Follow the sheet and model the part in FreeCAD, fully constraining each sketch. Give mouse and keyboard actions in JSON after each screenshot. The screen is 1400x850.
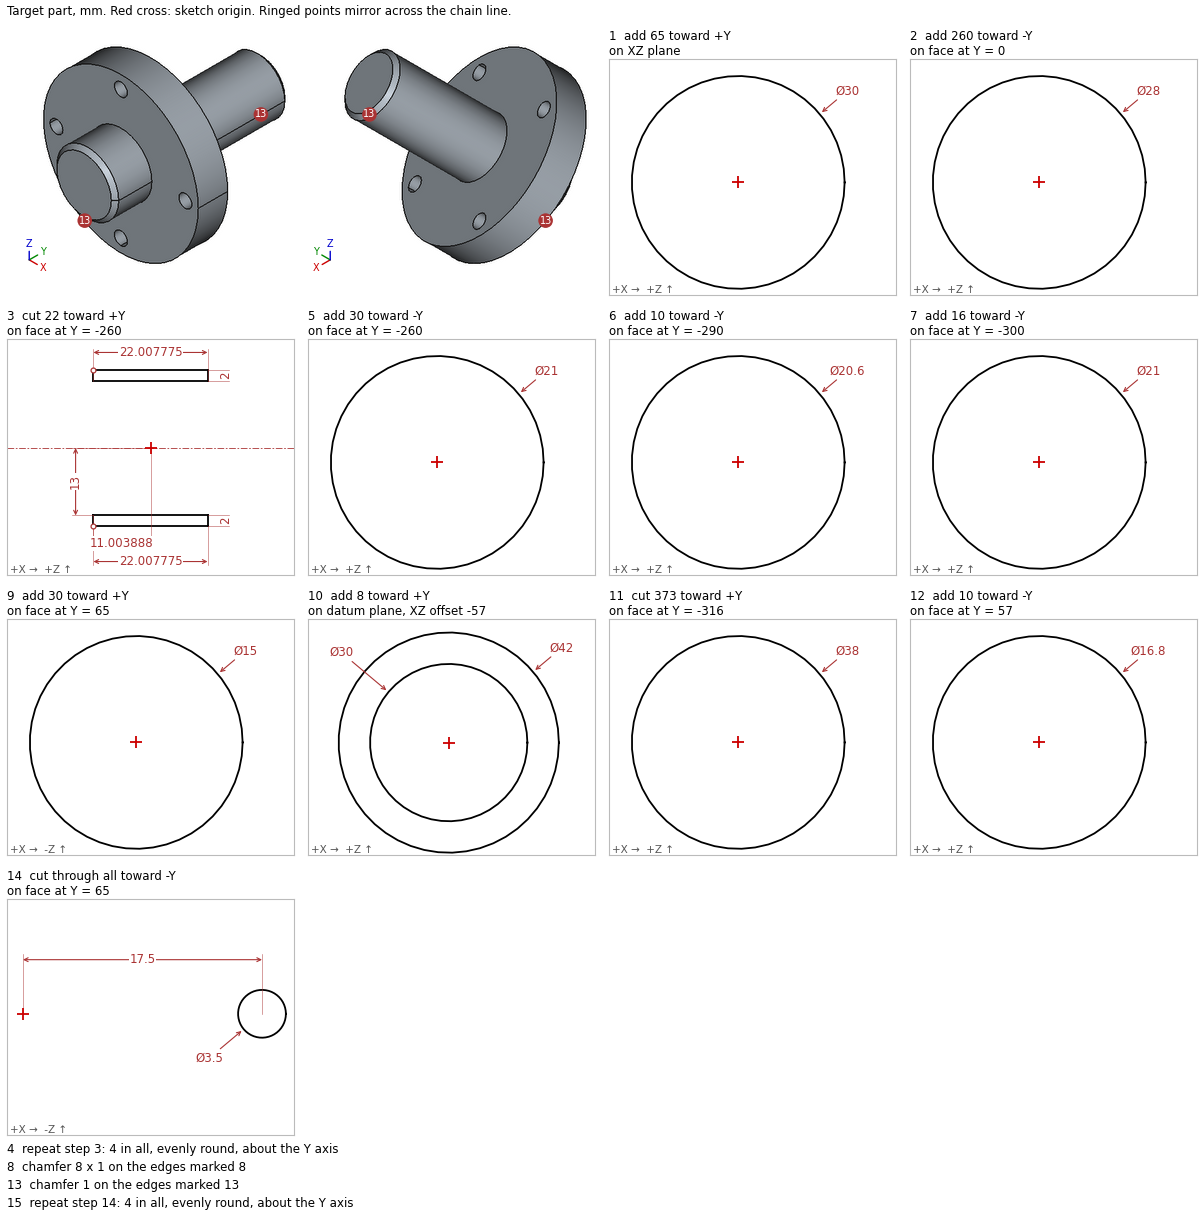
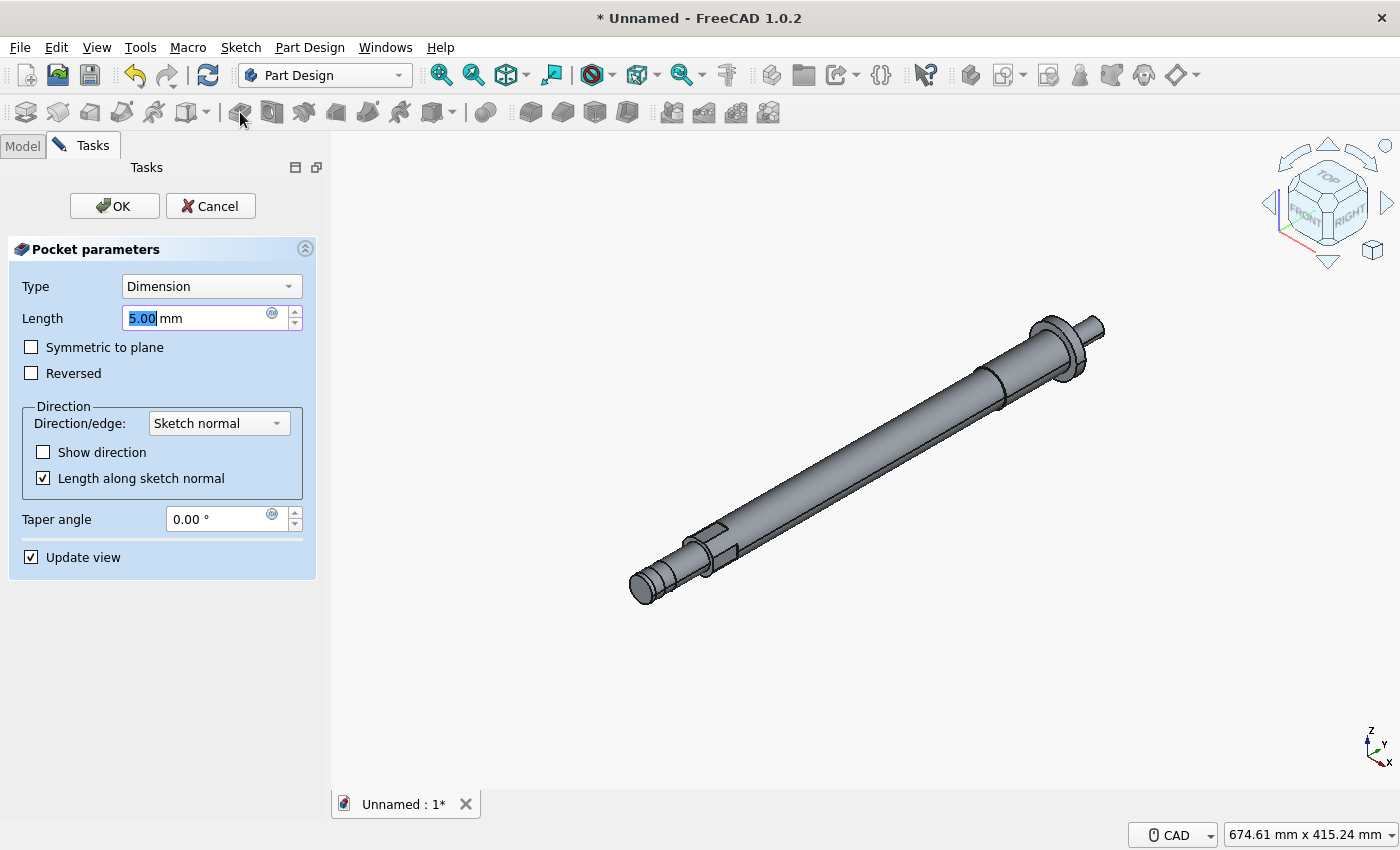
{"action": "type", "text": "373"}
{"action": "key", "text": "Tab"}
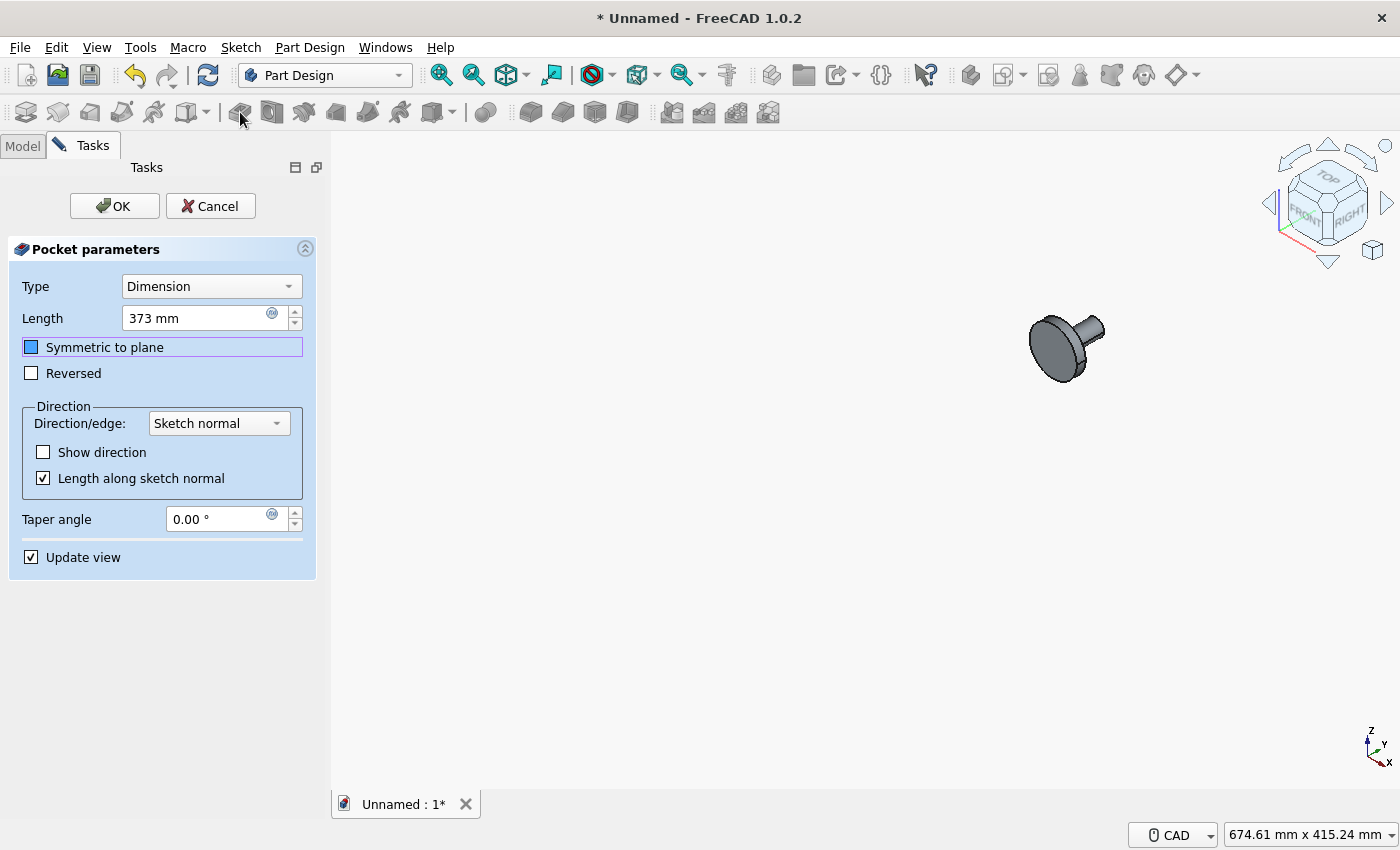
{"action": "left_click", "coordinate": [115, 206]}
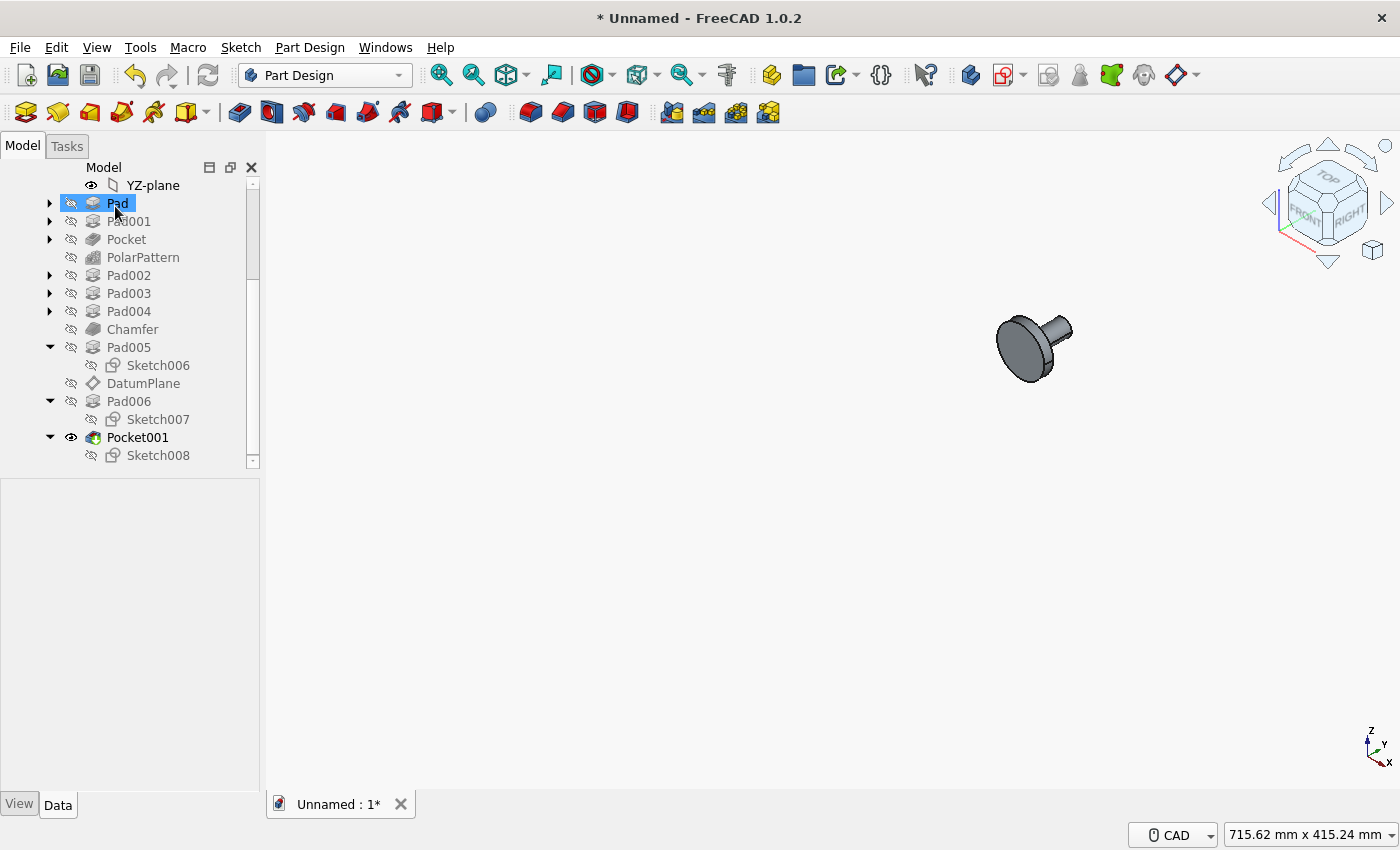
{"action": "left_click", "coordinate": [442, 76]}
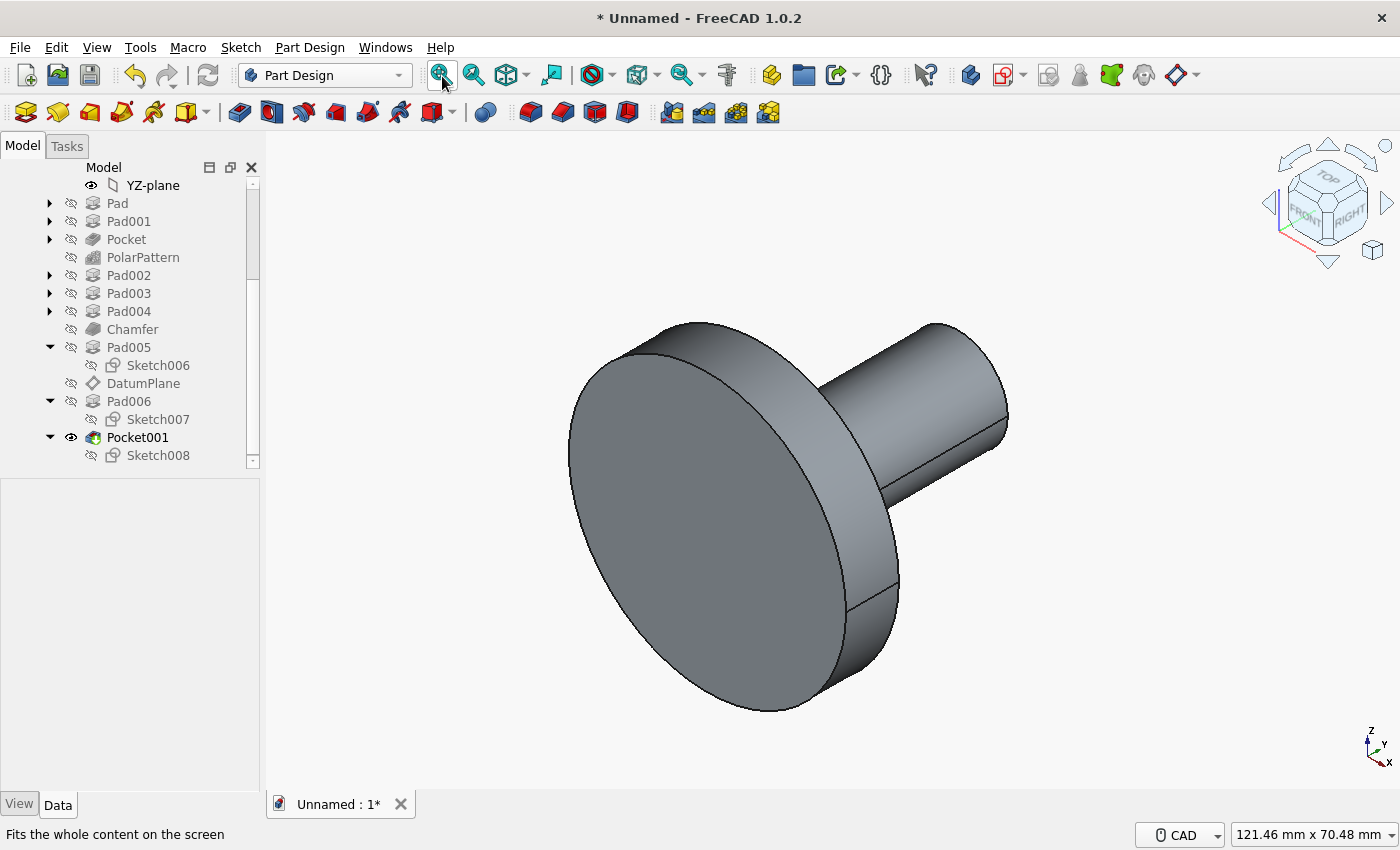
{"action": "left_click", "coordinate": [707, 531]}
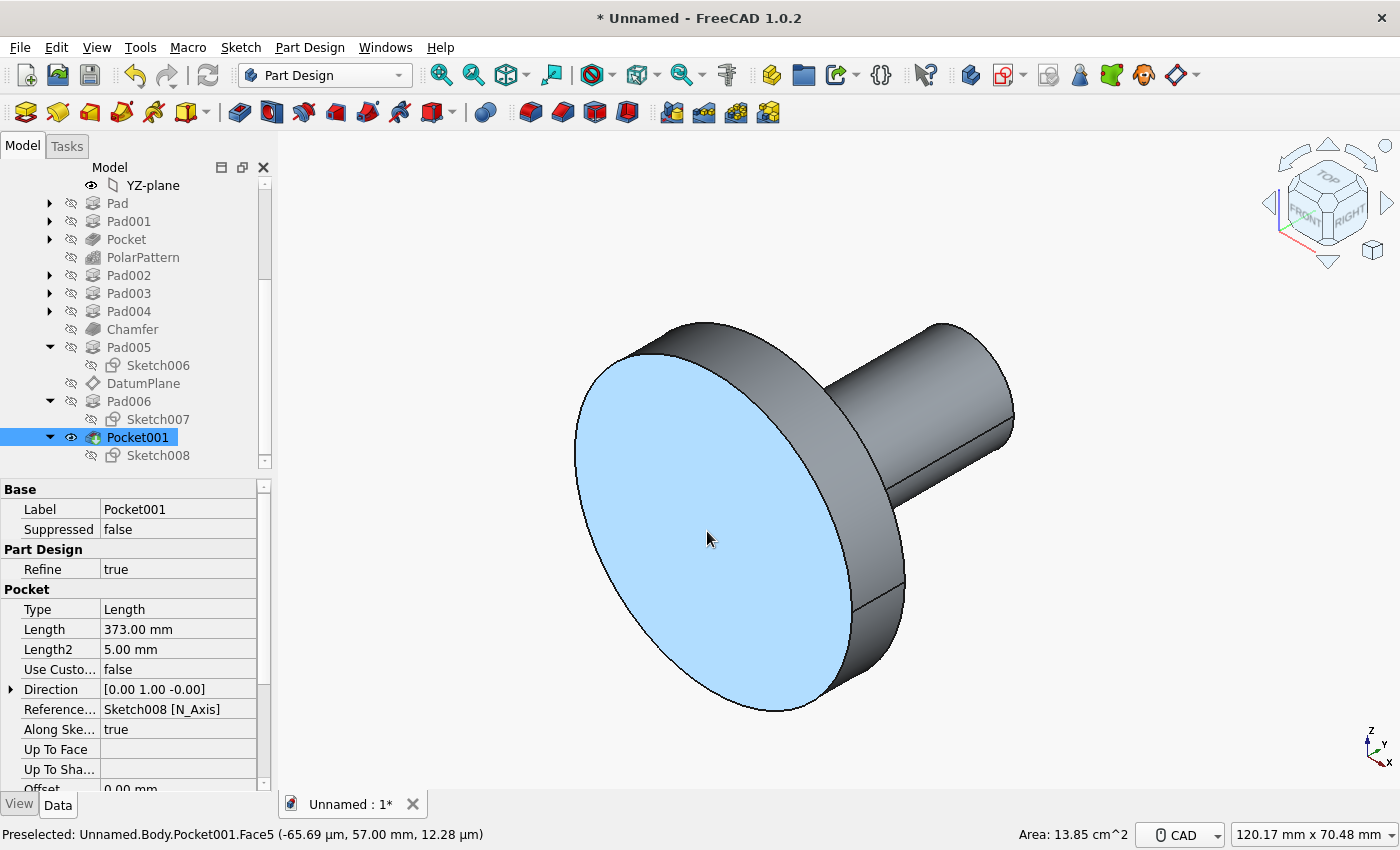
{"action": "left_click", "coordinate": [1004, 76]}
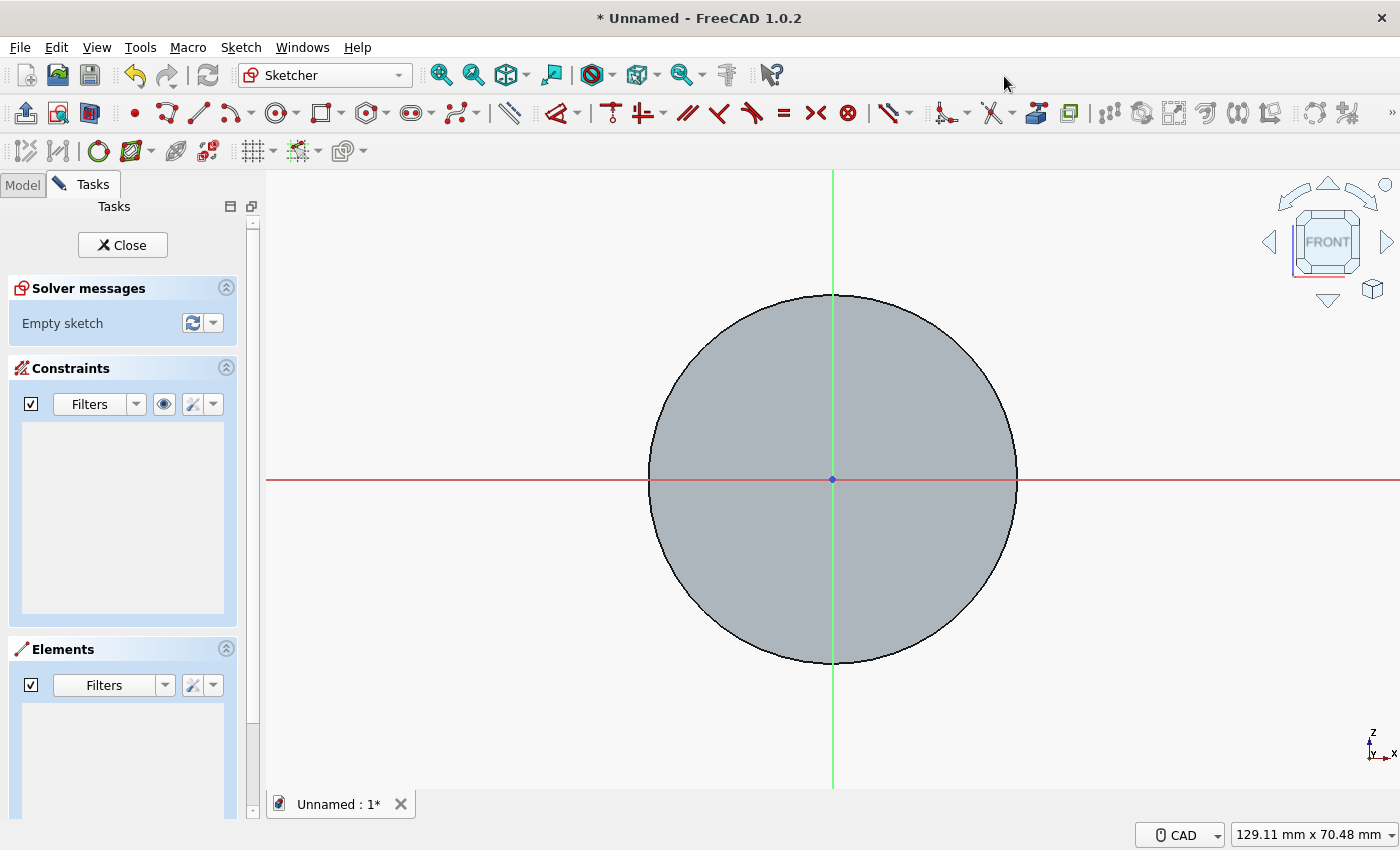
{"action": "scroll", "coordinate": [873, 480], "scroll_direction": "up", "scroll_amount": 5}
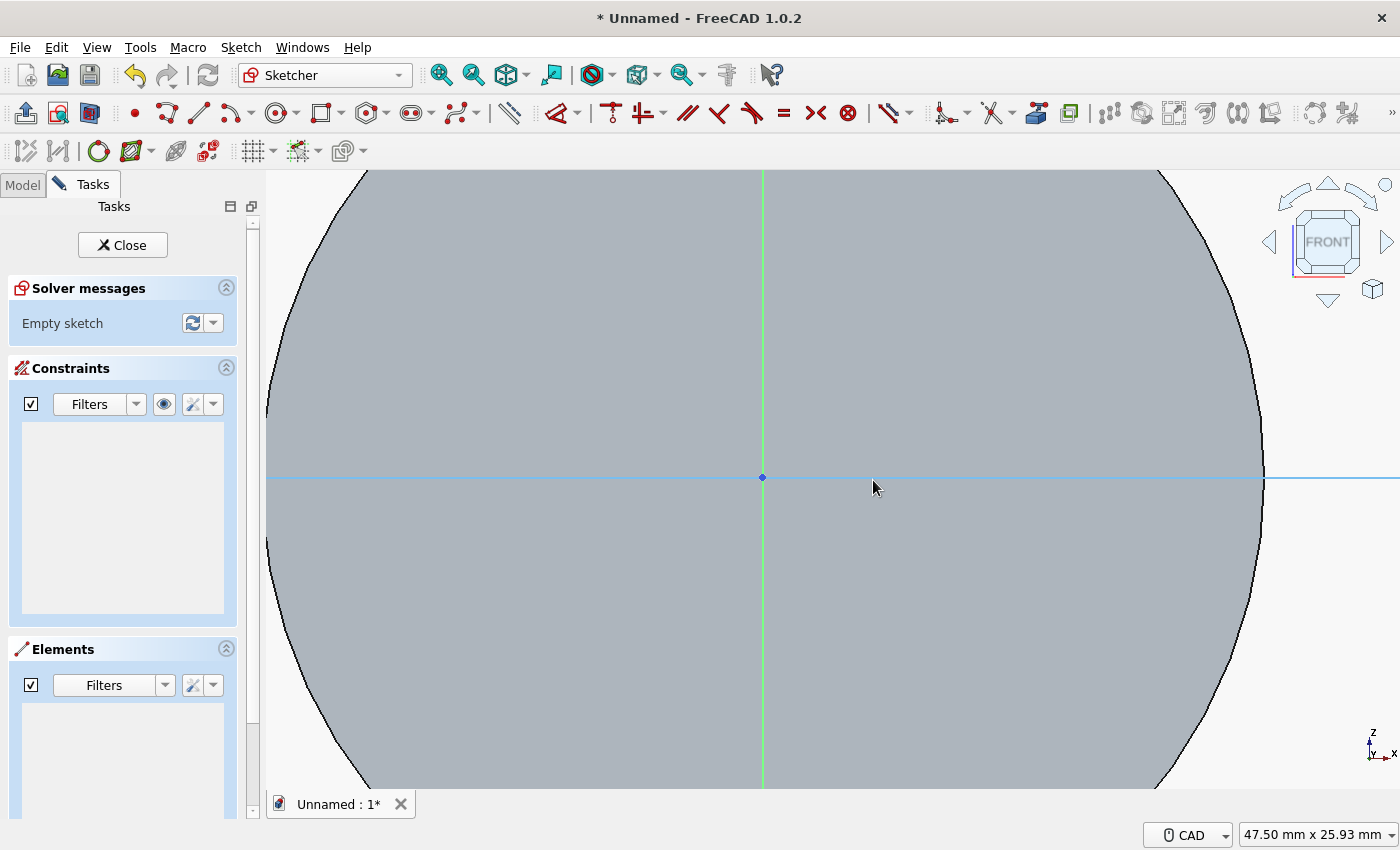
{"action": "left_click", "coordinate": [276, 114]}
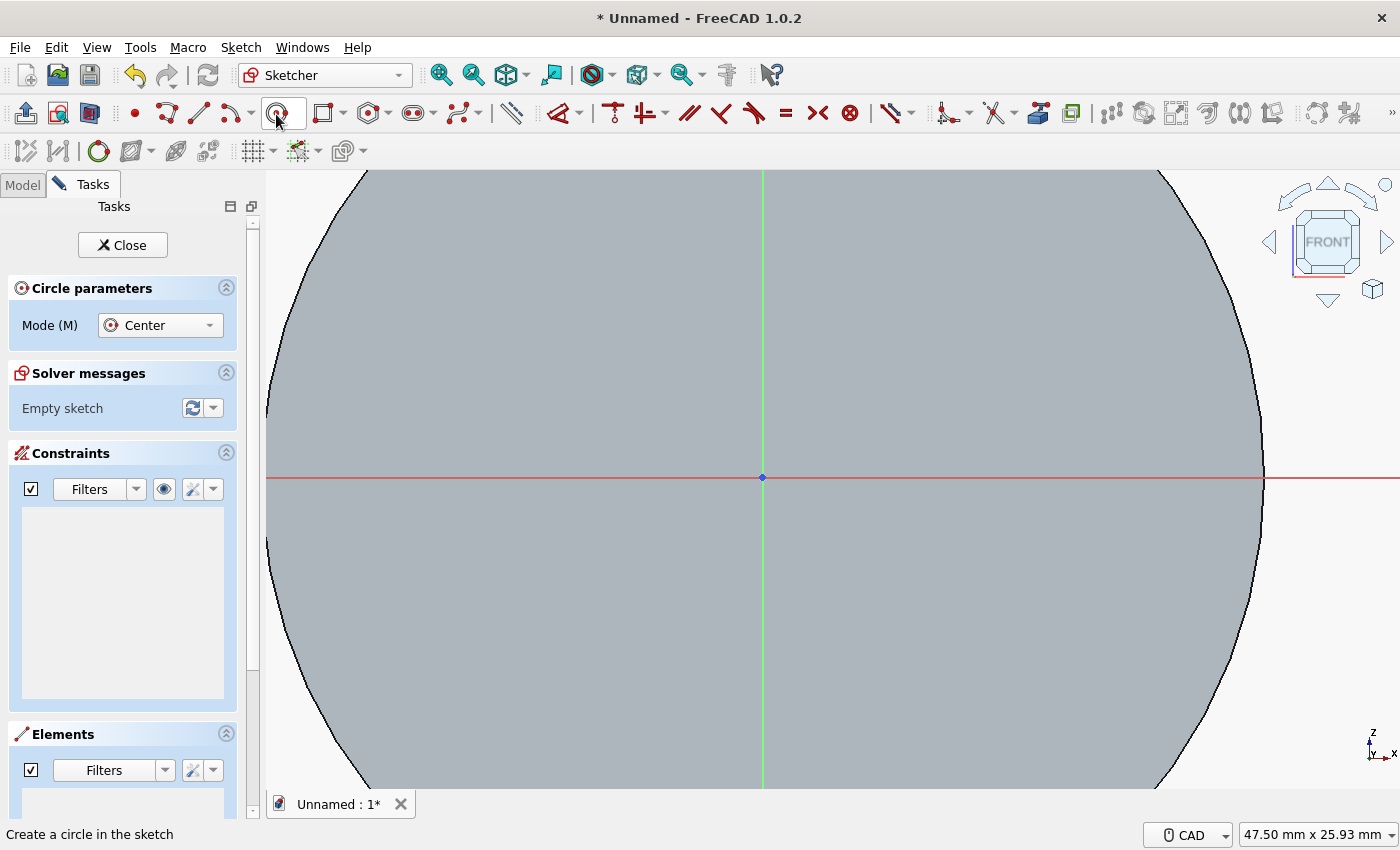
{"action": "left_click", "coordinate": [763, 478]}
{"action": "mouse_move", "coordinate": [905, 336]}